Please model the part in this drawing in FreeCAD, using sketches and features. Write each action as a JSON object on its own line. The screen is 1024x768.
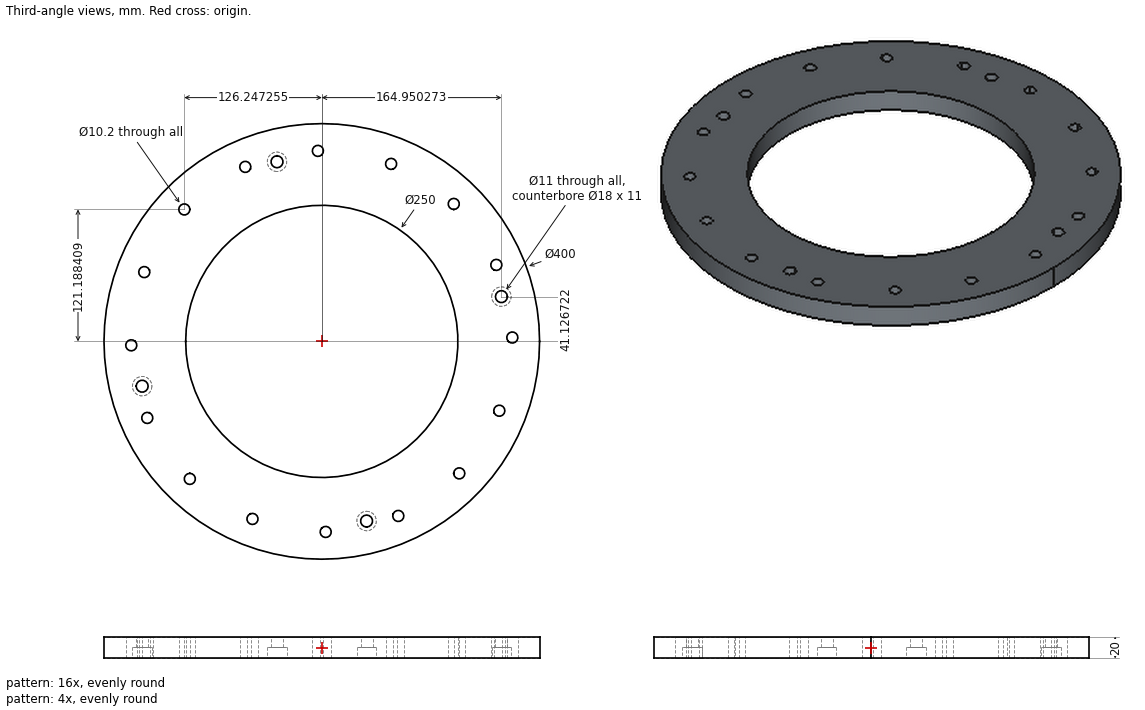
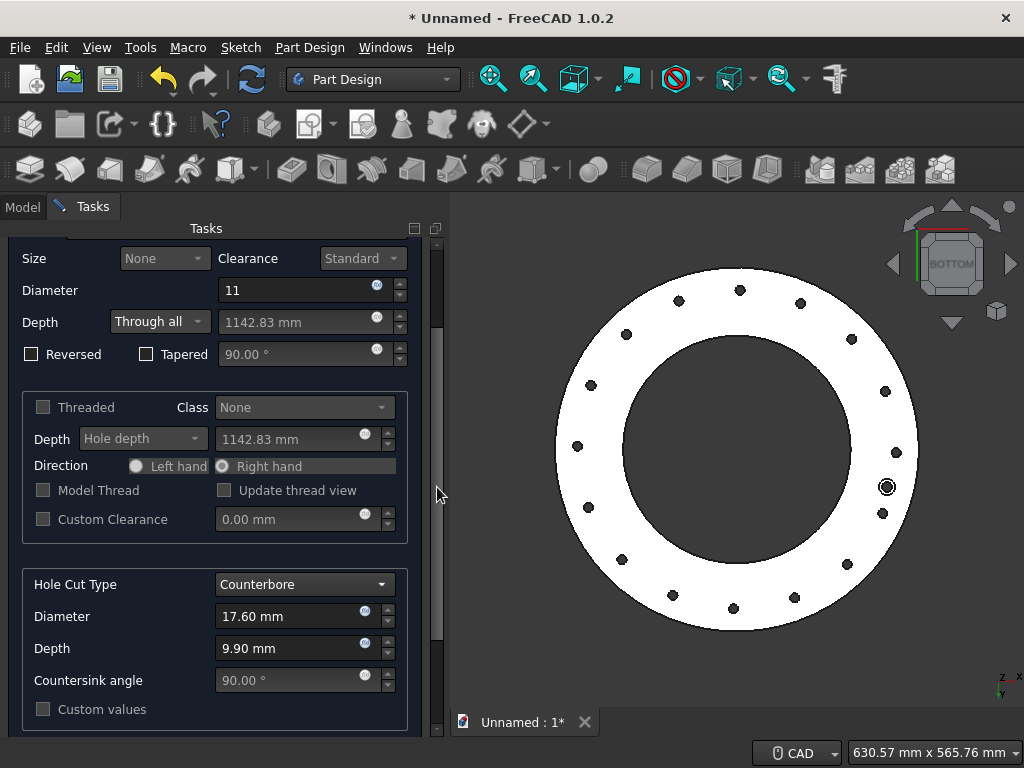
{"action": "triple_click", "coordinate": [298, 616]}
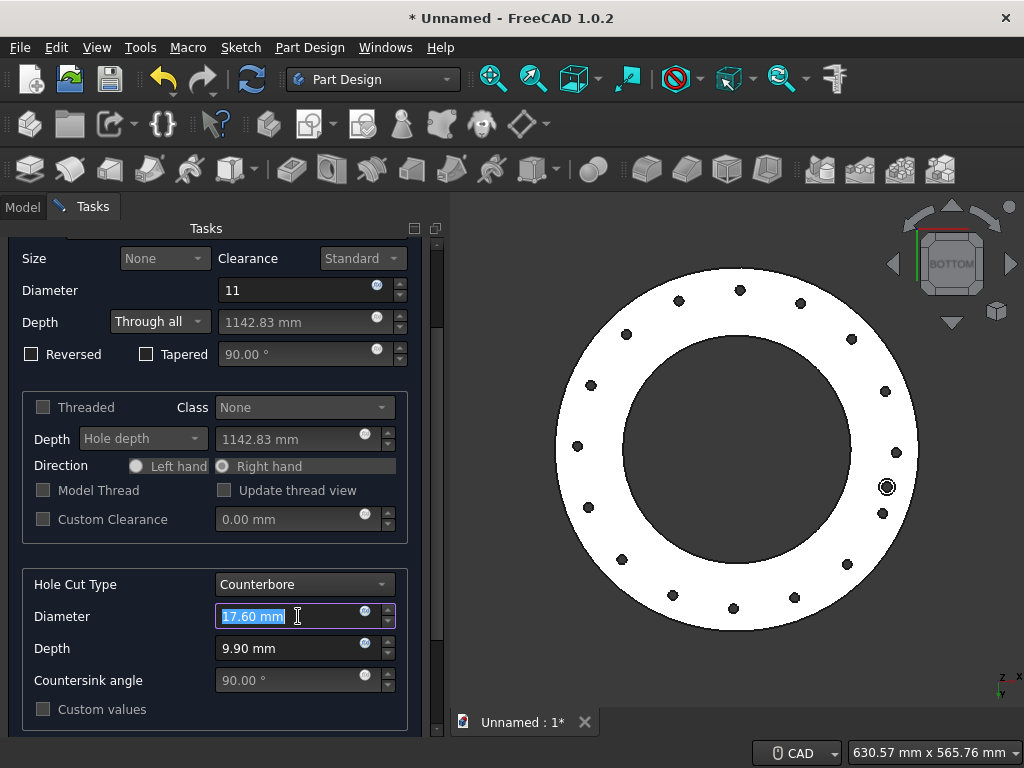
{"action": "type", "text": "18"}
{"action": "key", "text": "Tab"}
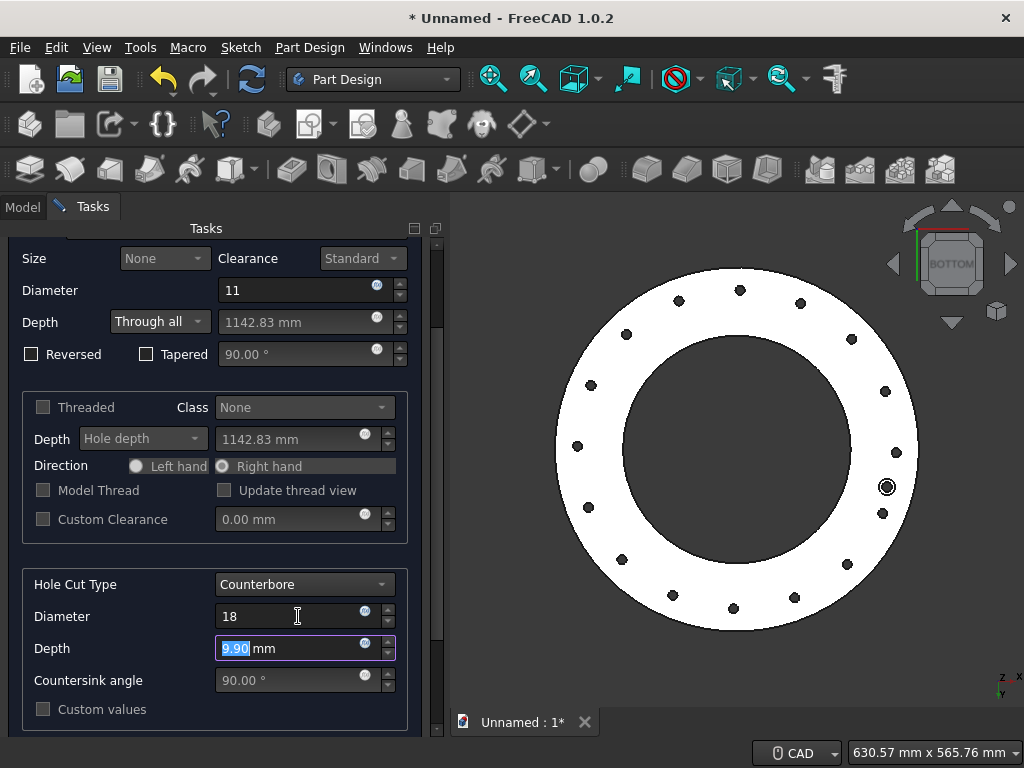
{"action": "type", "text": "11"}
{"action": "key", "text": "Tab"}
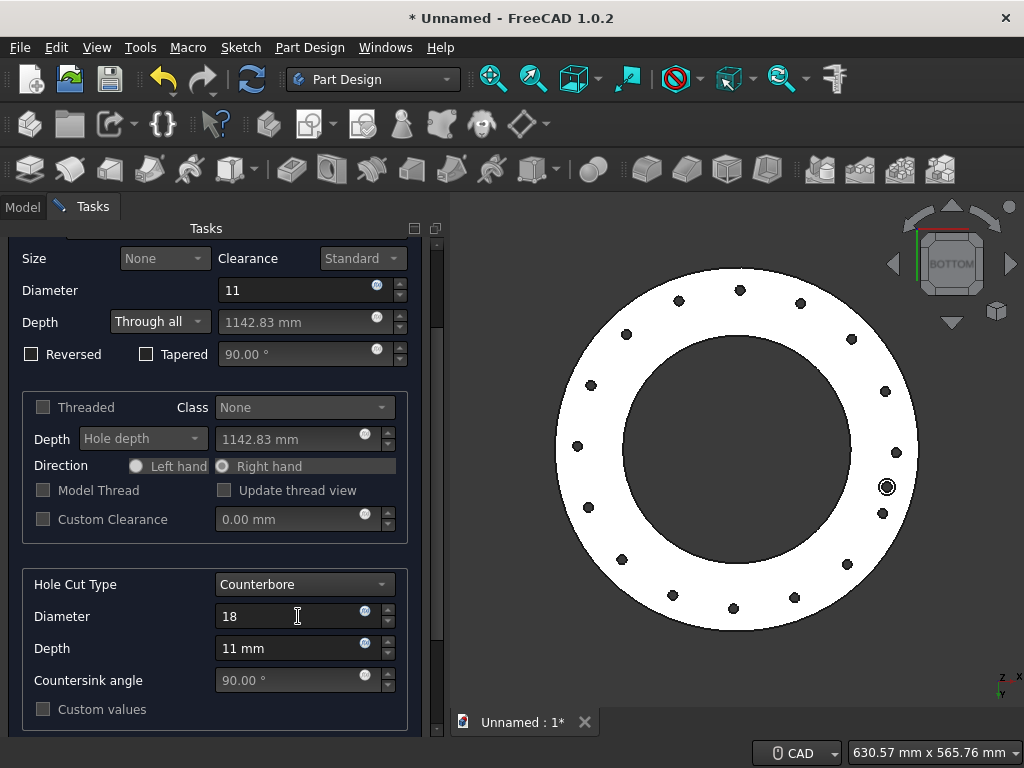
{"action": "scroll", "coordinate": [437, 487], "scroll_direction": "up", "scroll_amount": 3}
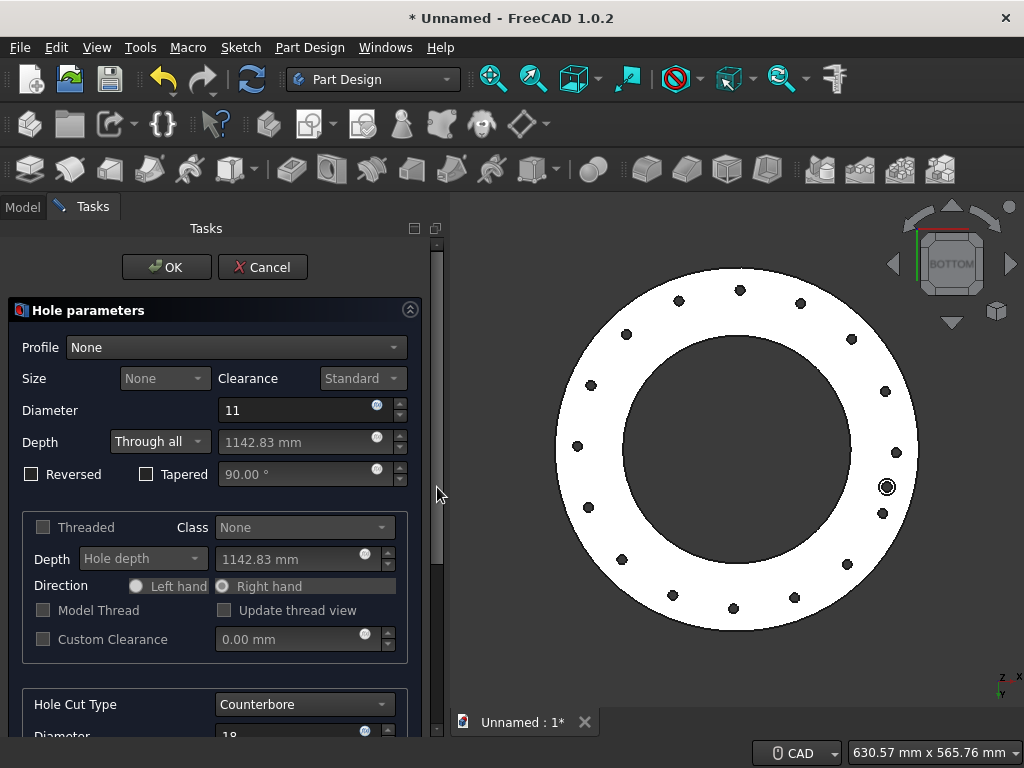
{"action": "left_click", "coordinate": [167, 267]}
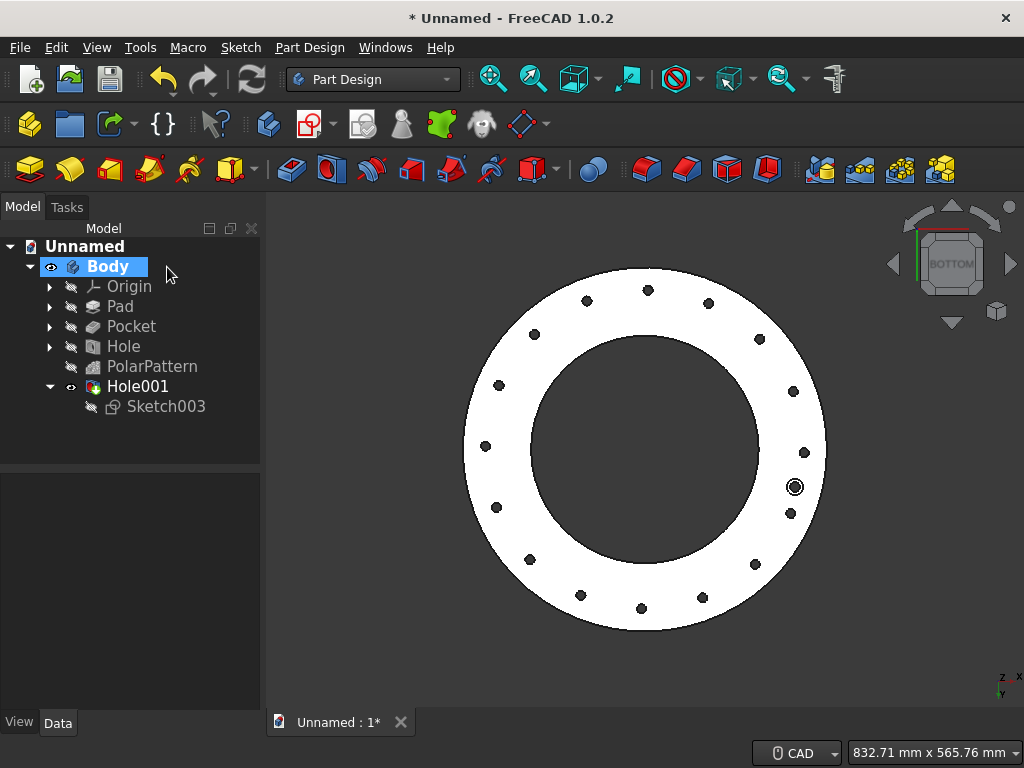
{"action": "left_click", "coordinate": [116, 387]}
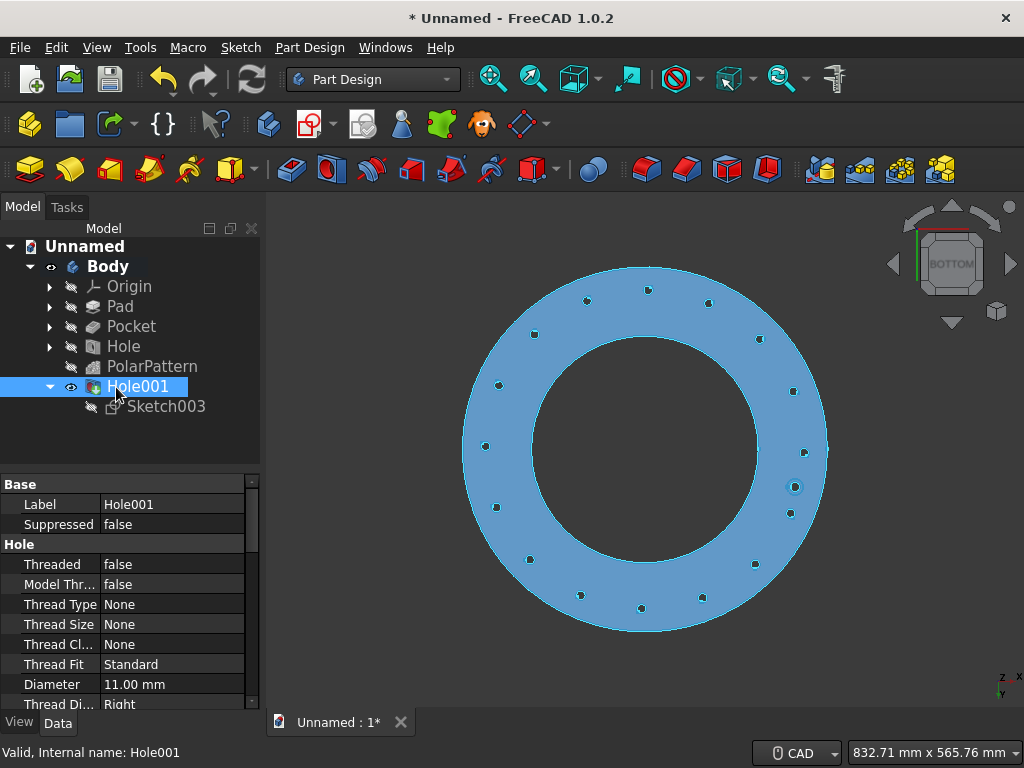
{"action": "left_click", "coordinate": [900, 170]}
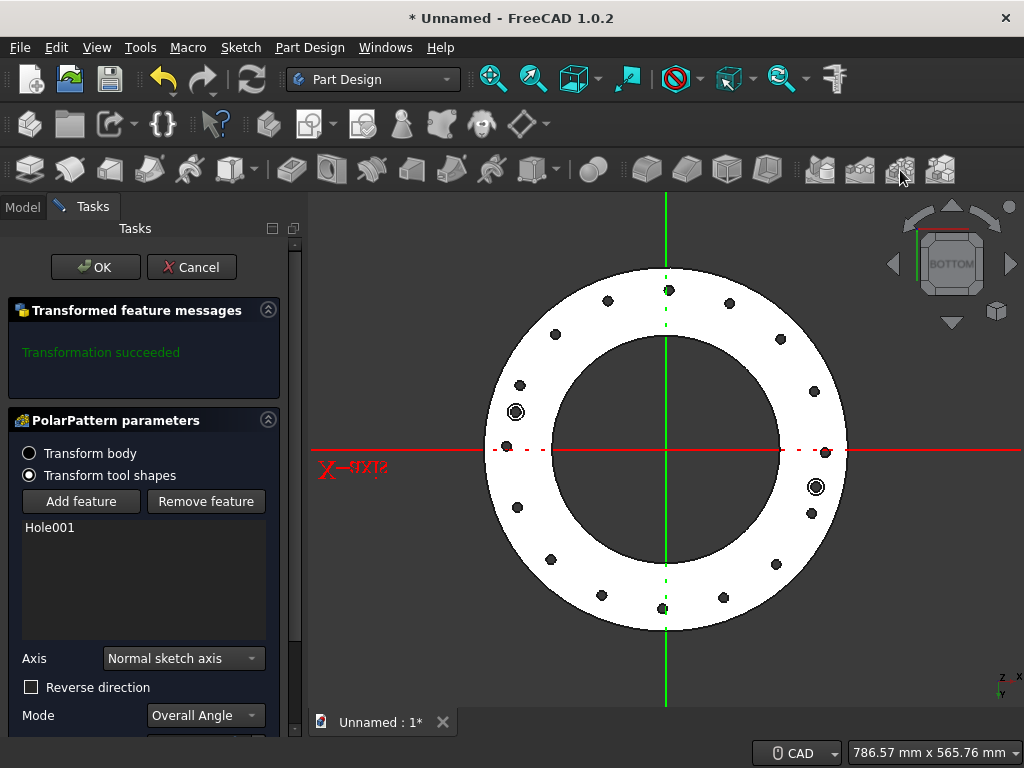
{"action": "left_click", "coordinate": [184, 658]}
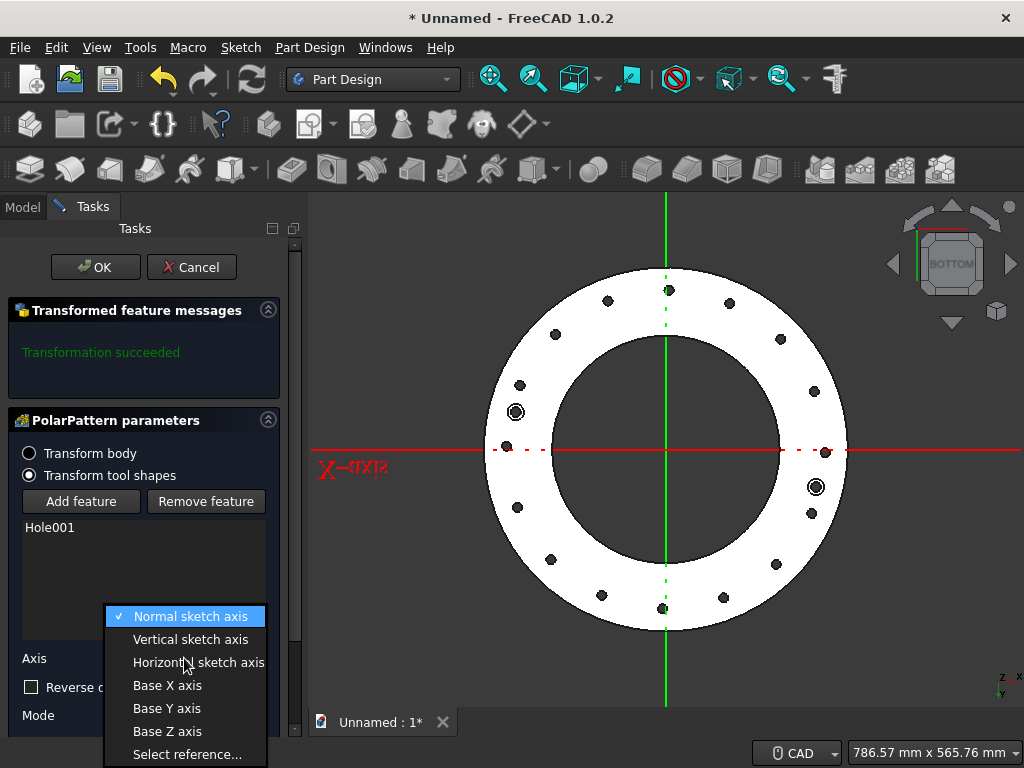
{"action": "left_click", "coordinate": [184, 732]}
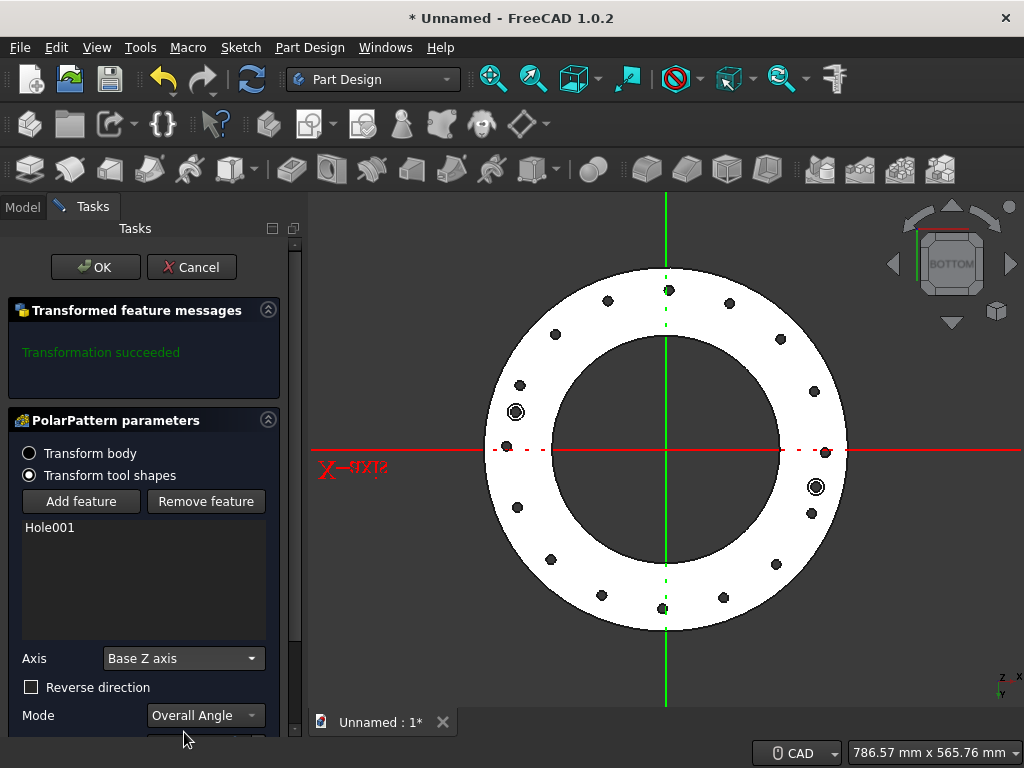
{"action": "scroll", "coordinate": [295, 487], "scroll_direction": "down", "scroll_amount": 2}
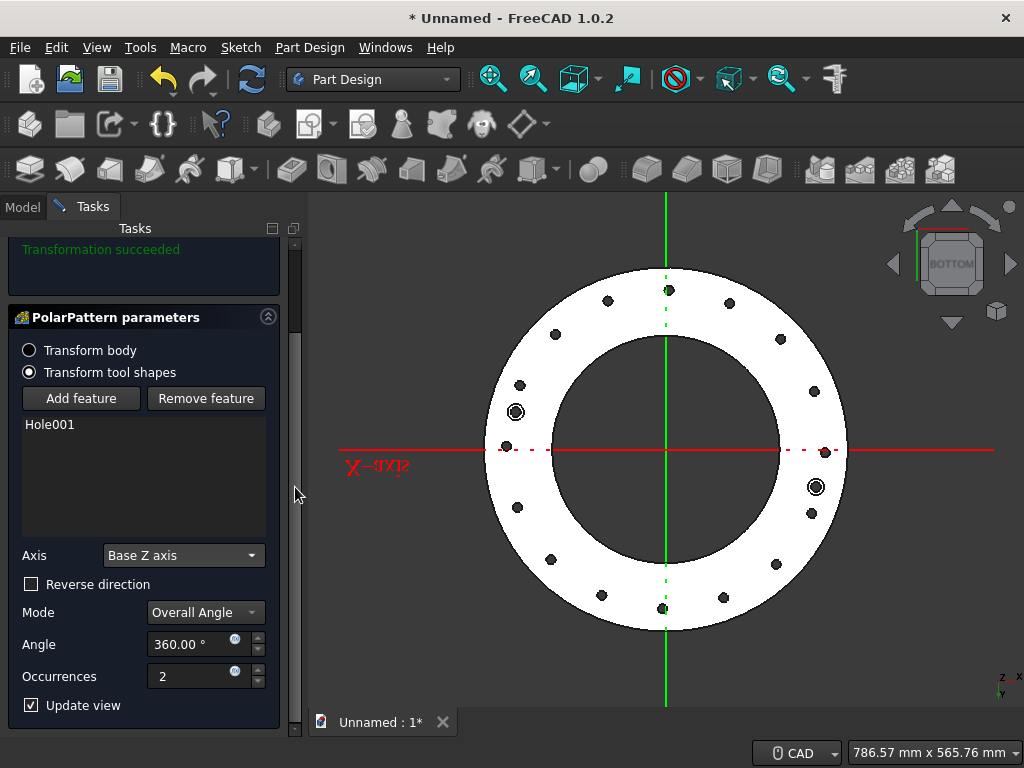
{"action": "triple_click", "coordinate": [198, 676]}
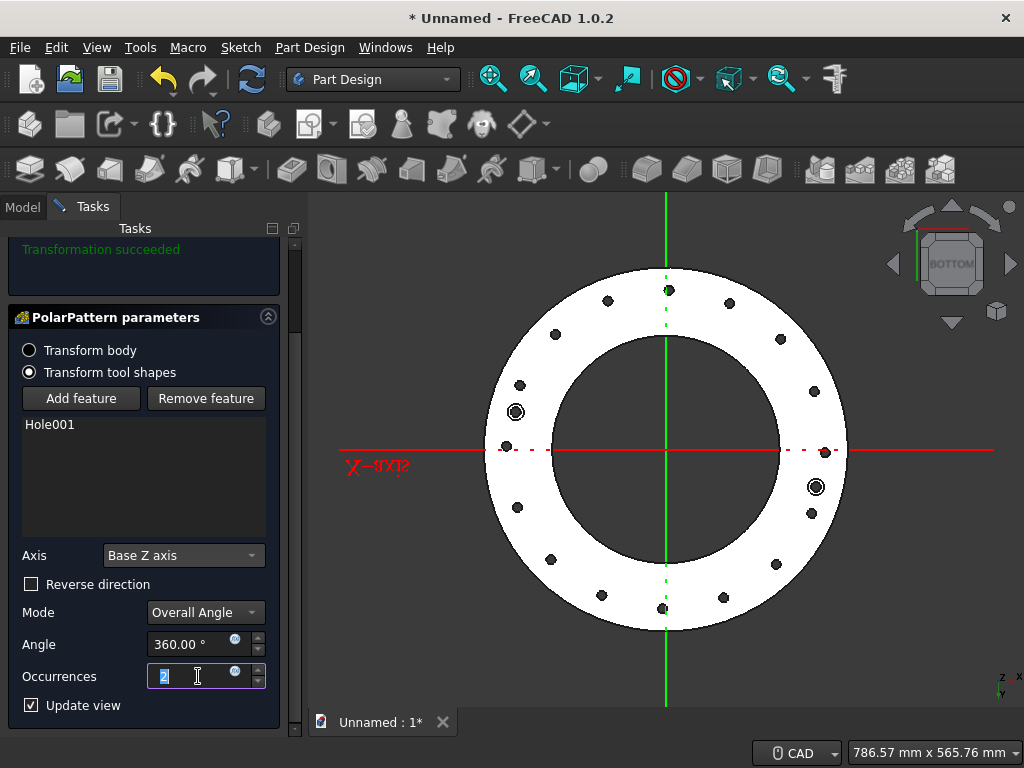
{"action": "type", "text": "4"}
{"action": "key", "text": "Tab"}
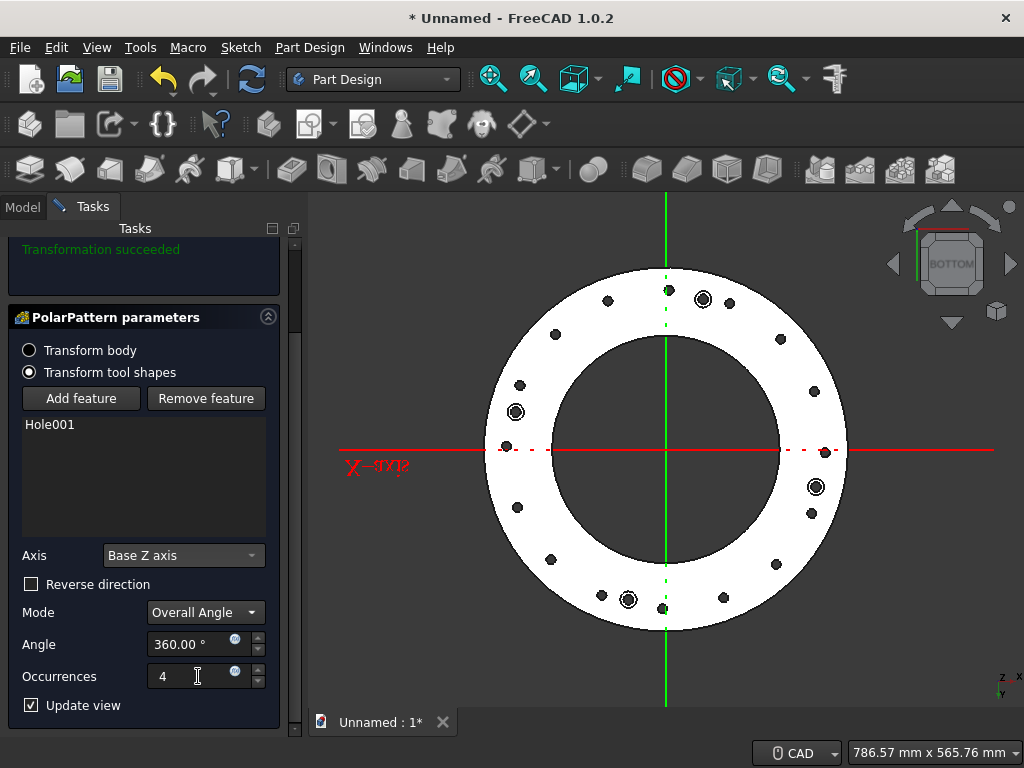
{"action": "scroll", "coordinate": [295, 487], "scroll_direction": "up", "scroll_amount": 3}